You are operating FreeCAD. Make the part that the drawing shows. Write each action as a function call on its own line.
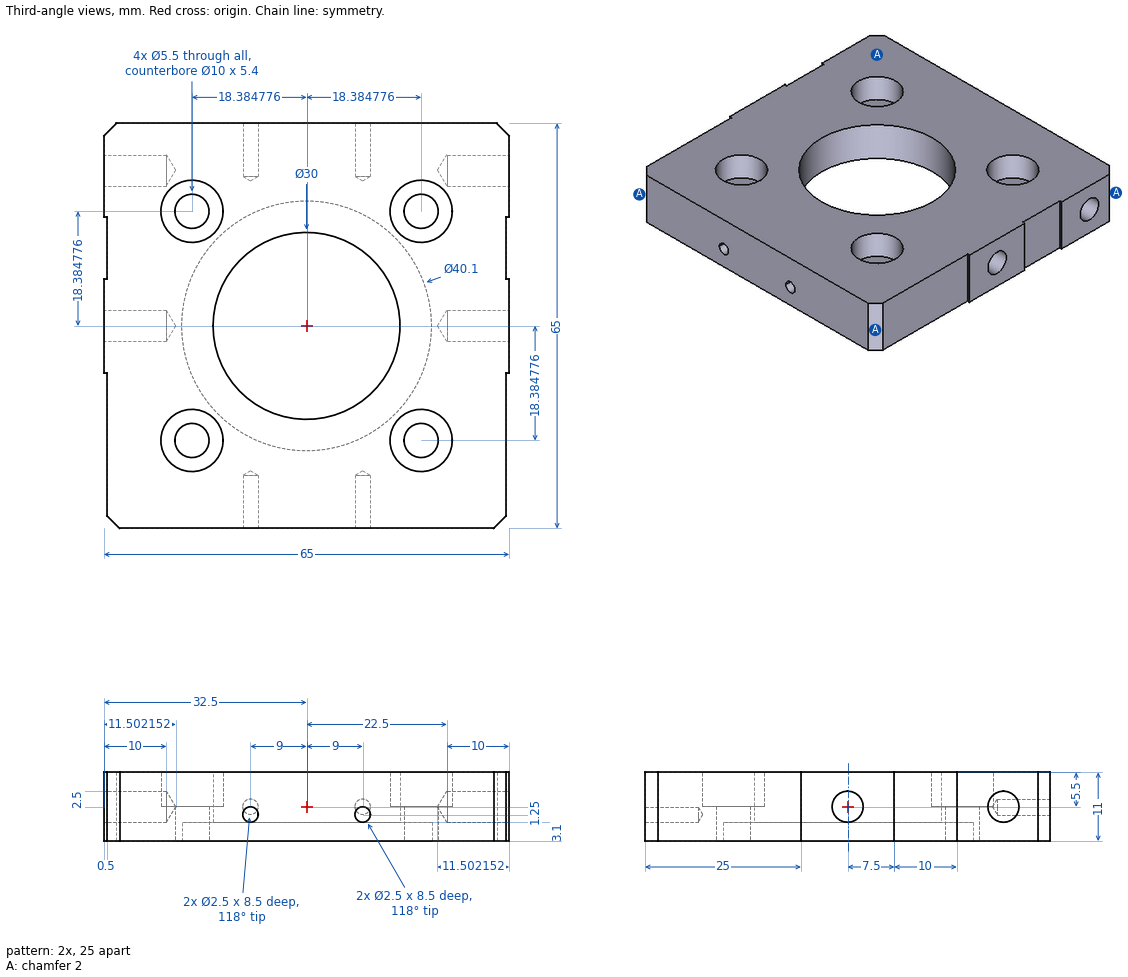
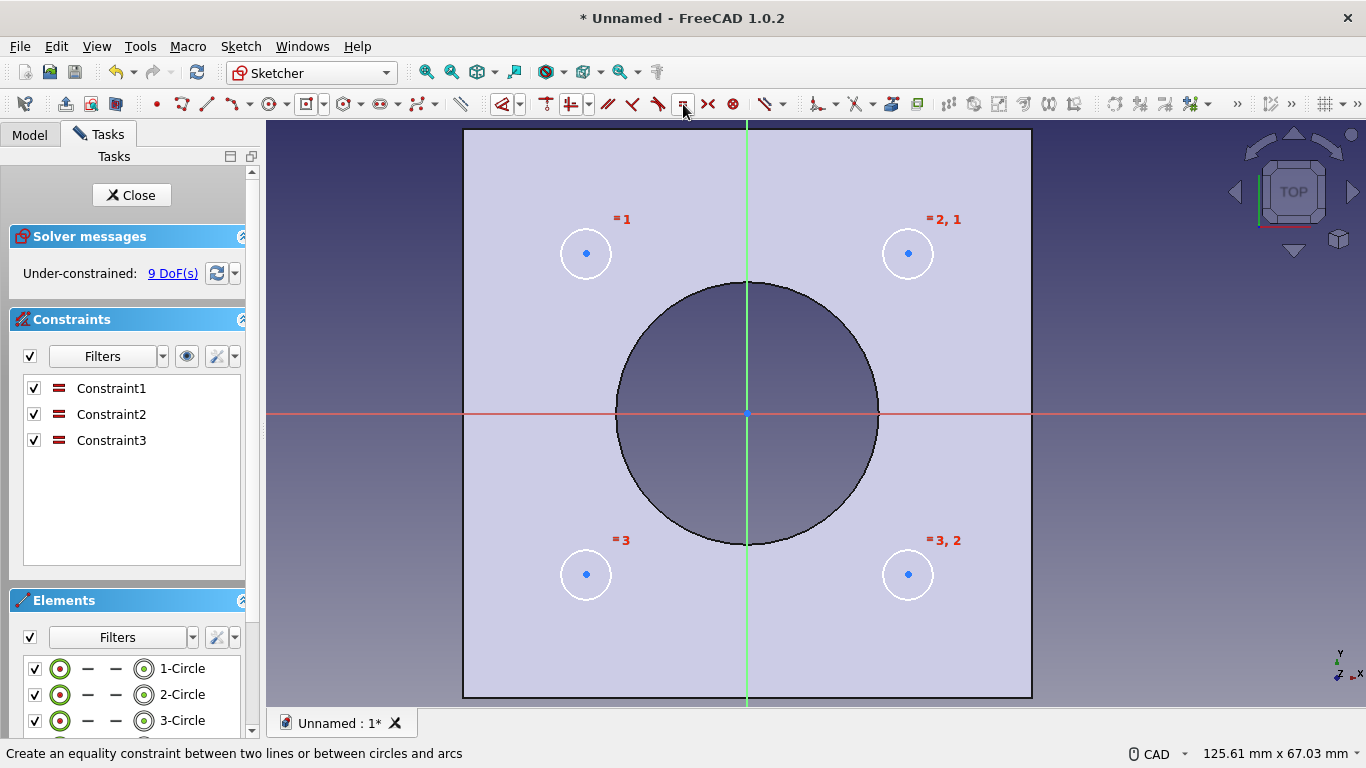
click(586, 254)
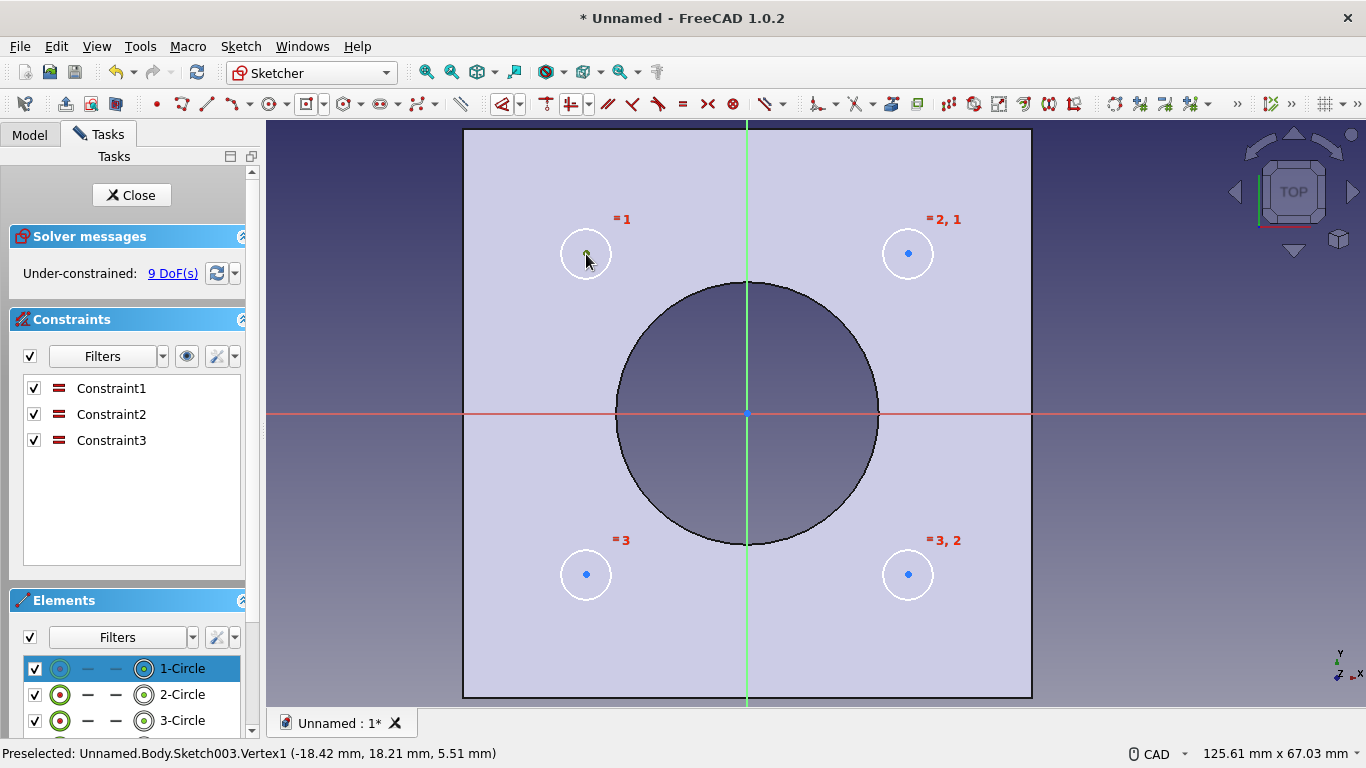
click(908, 254)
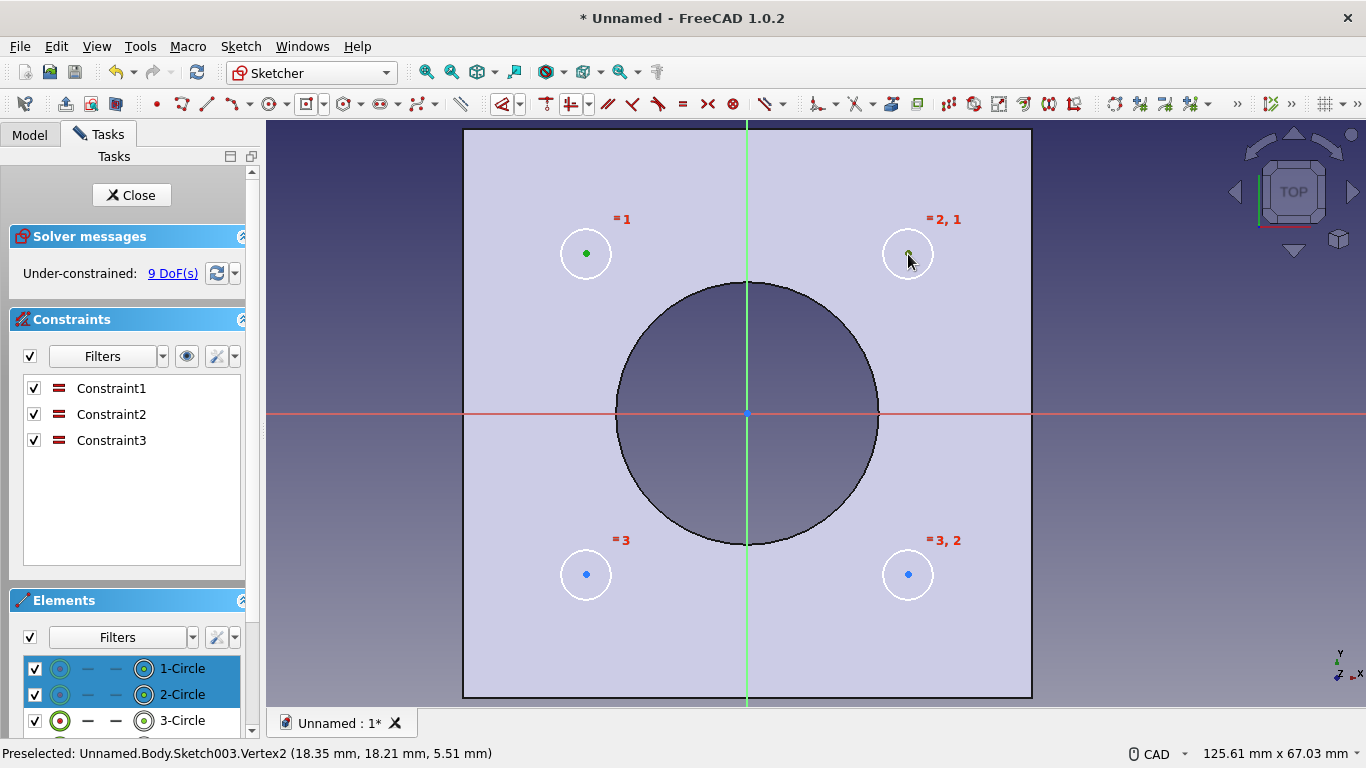
click(588, 104)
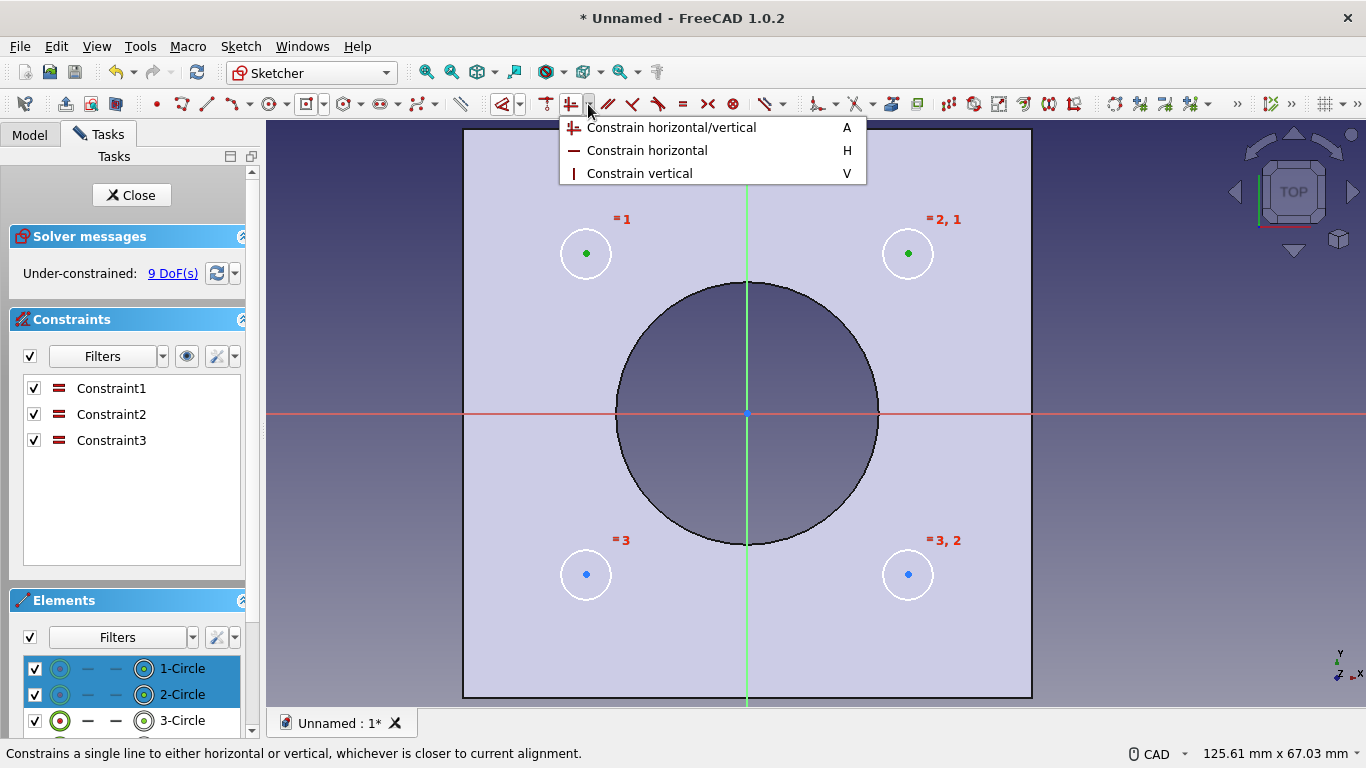
click(713, 150)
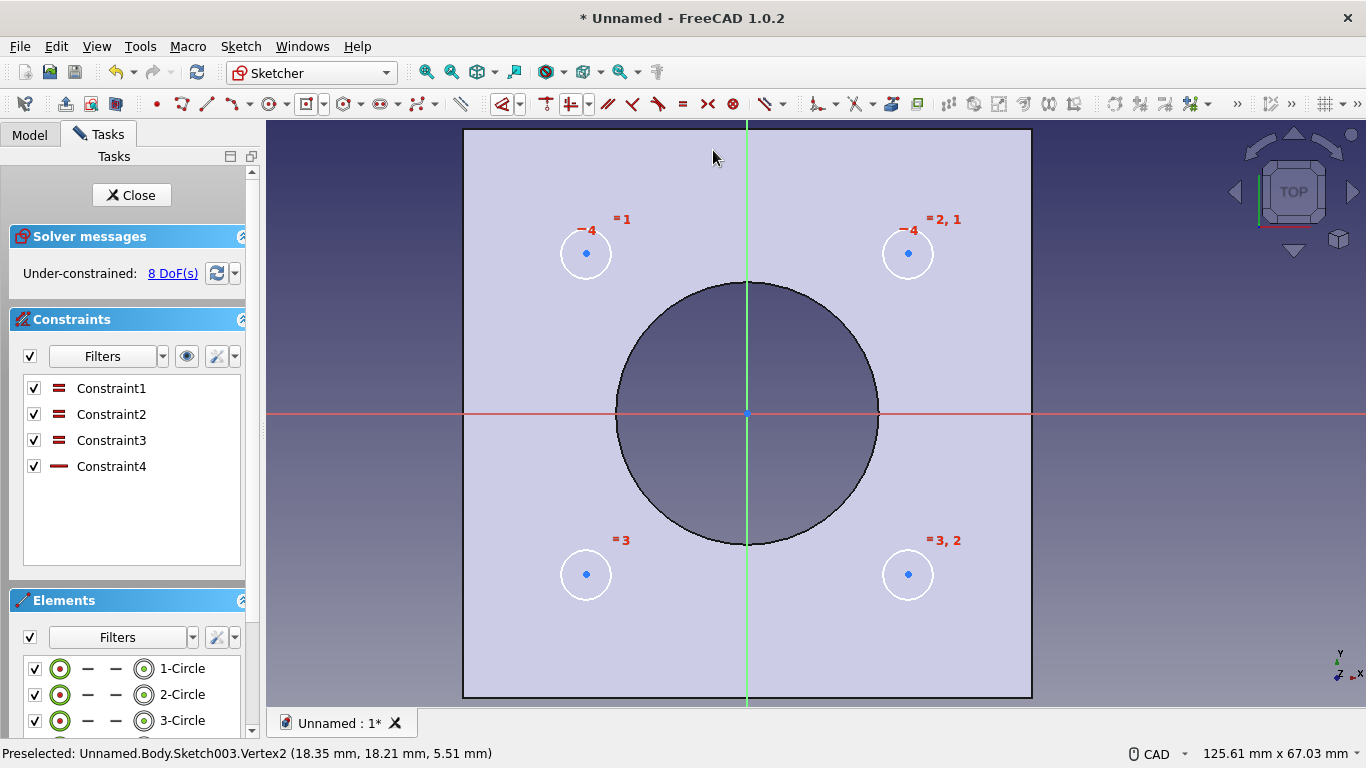
click(908, 254)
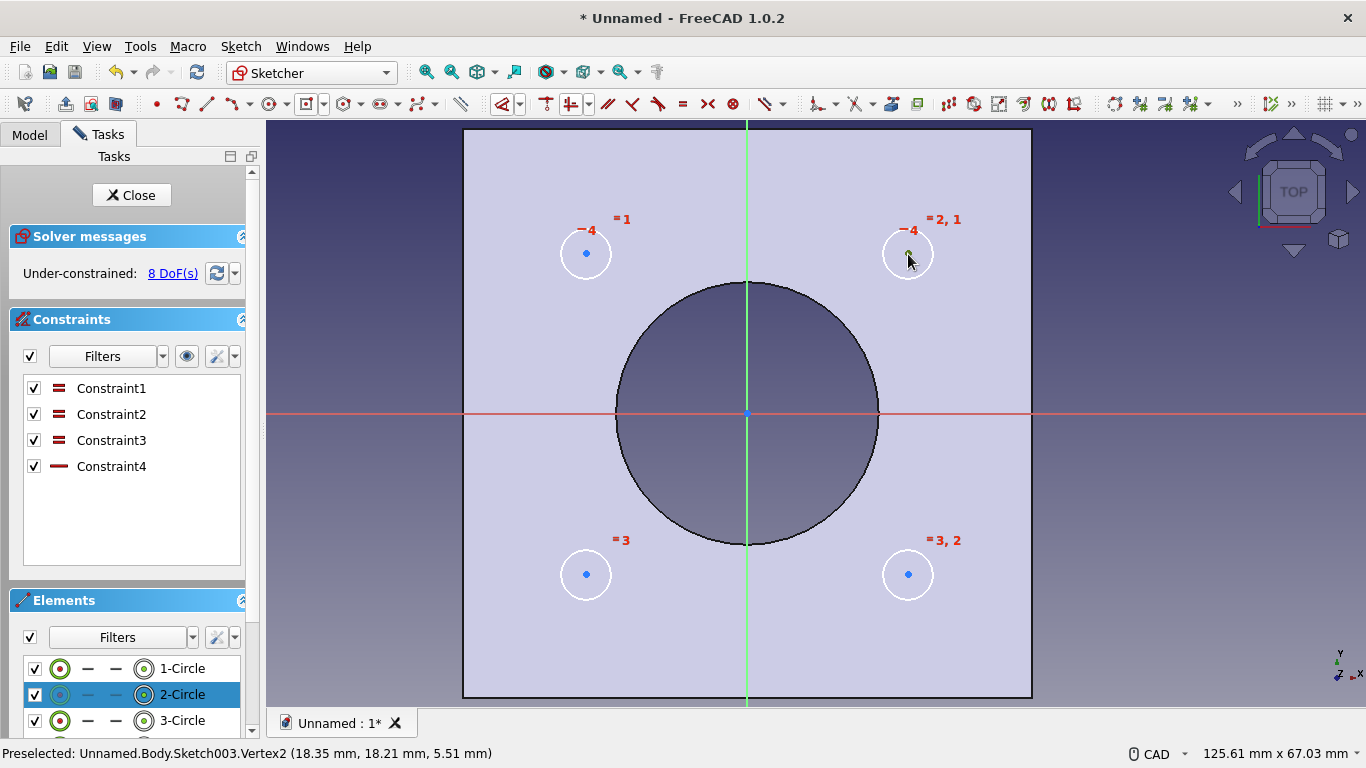
click(908, 575)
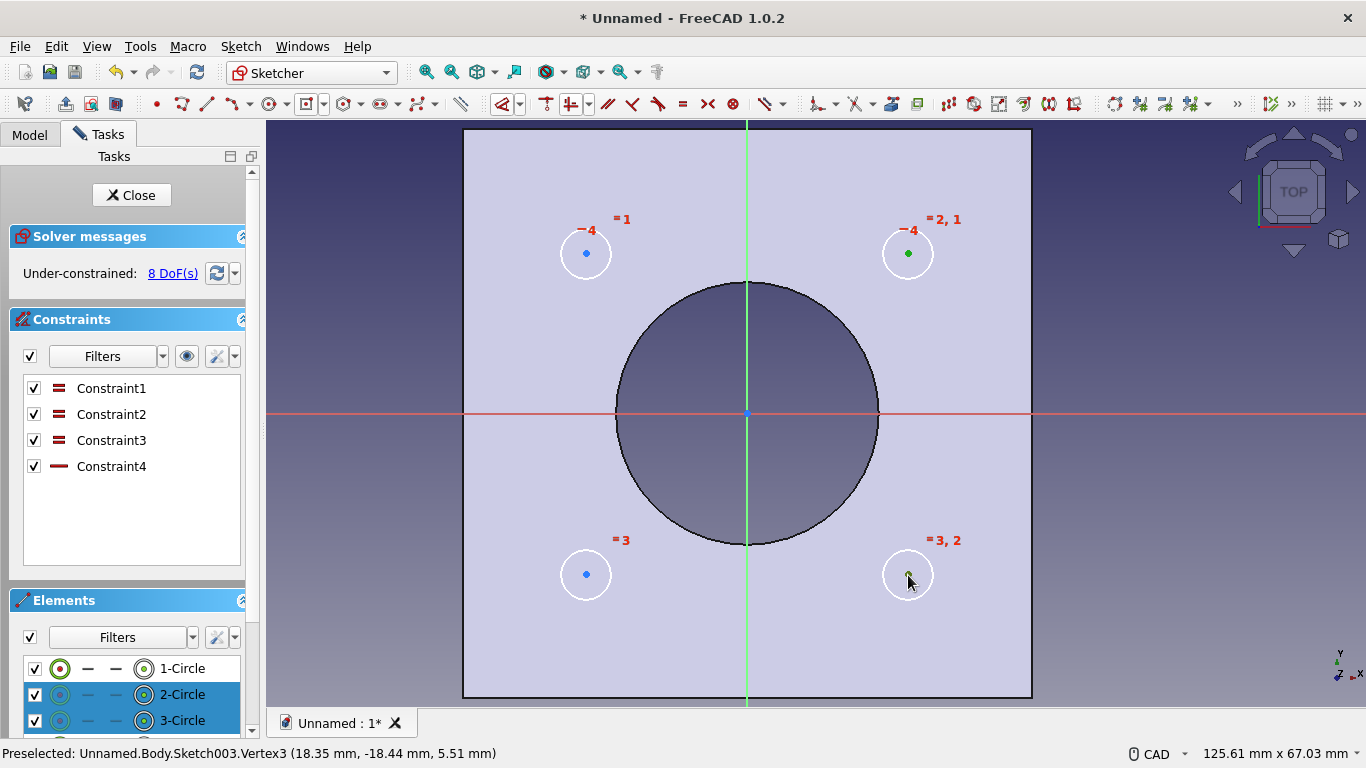
key(v)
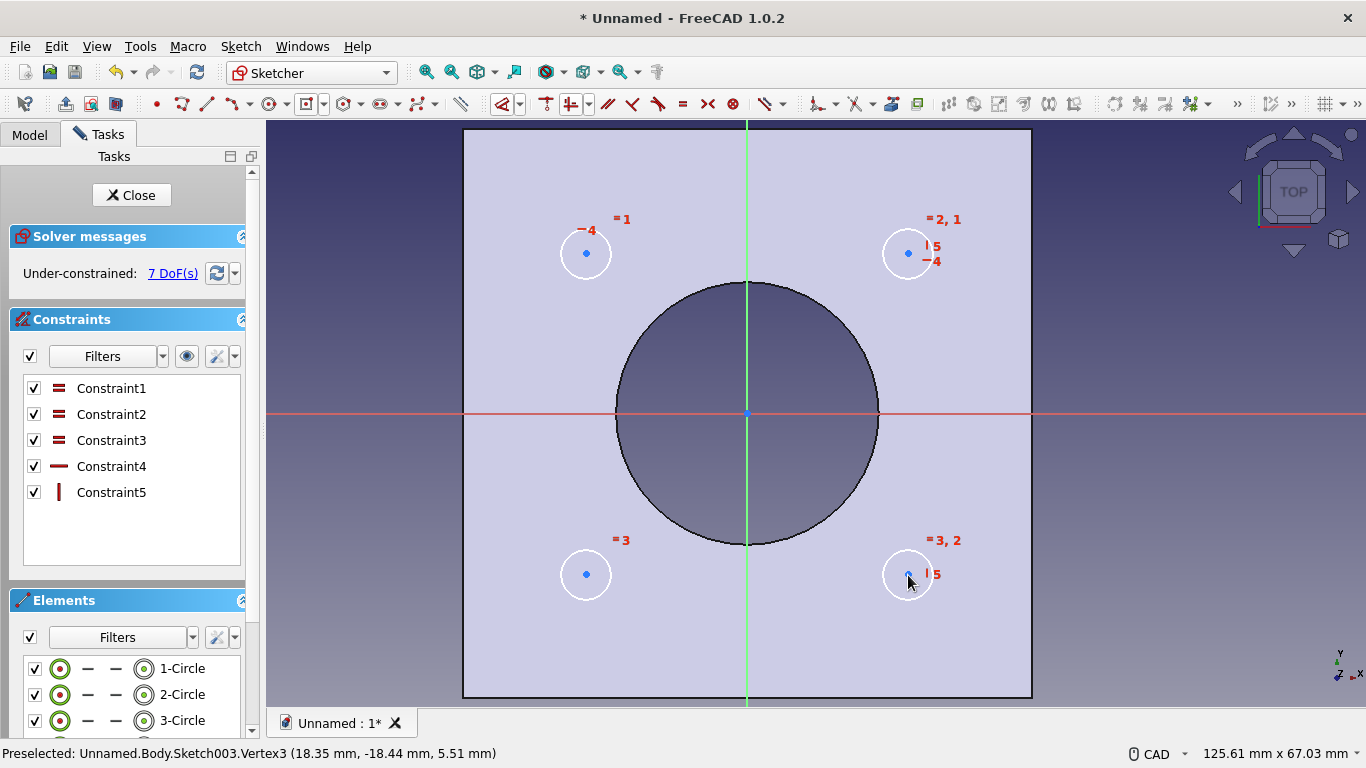
click(586, 254)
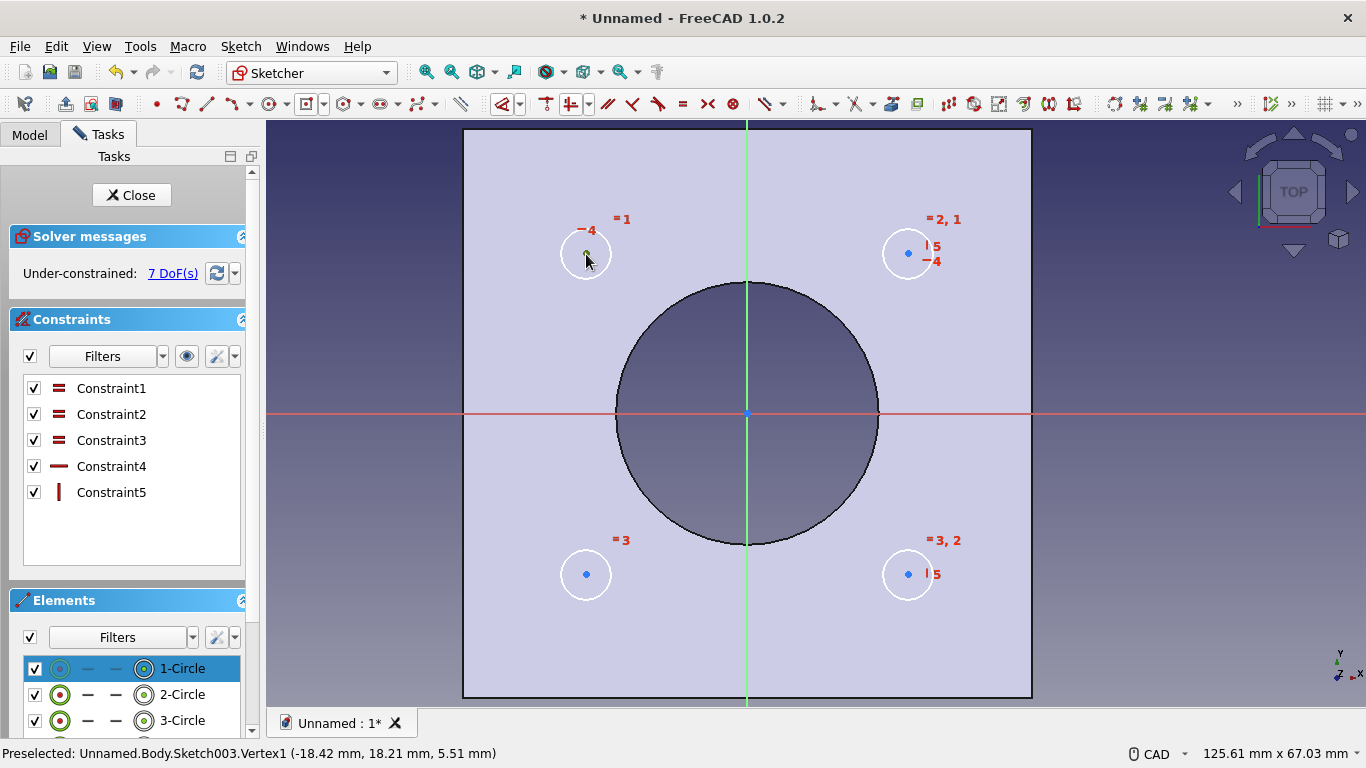
click(586, 575)